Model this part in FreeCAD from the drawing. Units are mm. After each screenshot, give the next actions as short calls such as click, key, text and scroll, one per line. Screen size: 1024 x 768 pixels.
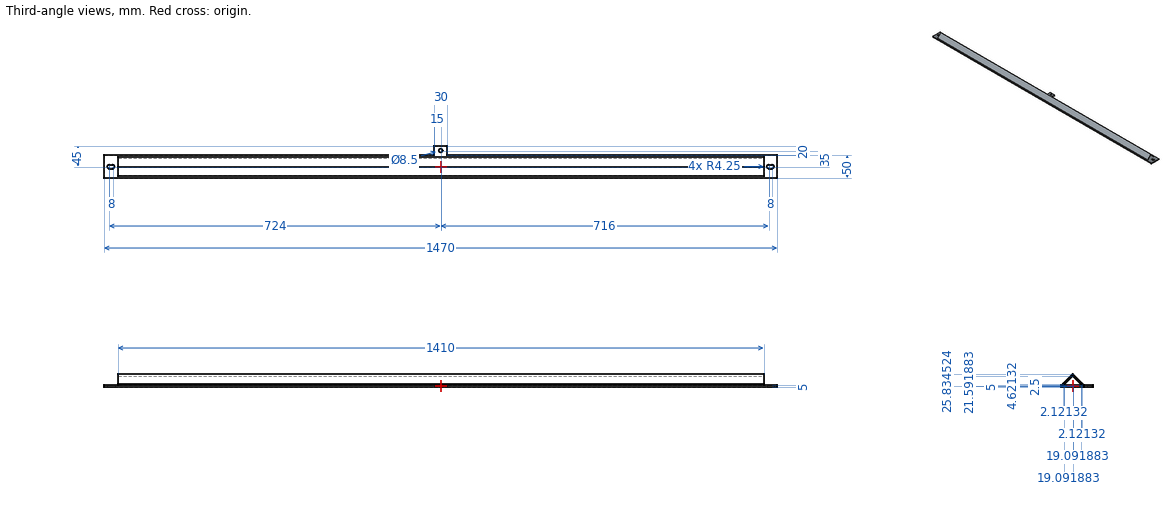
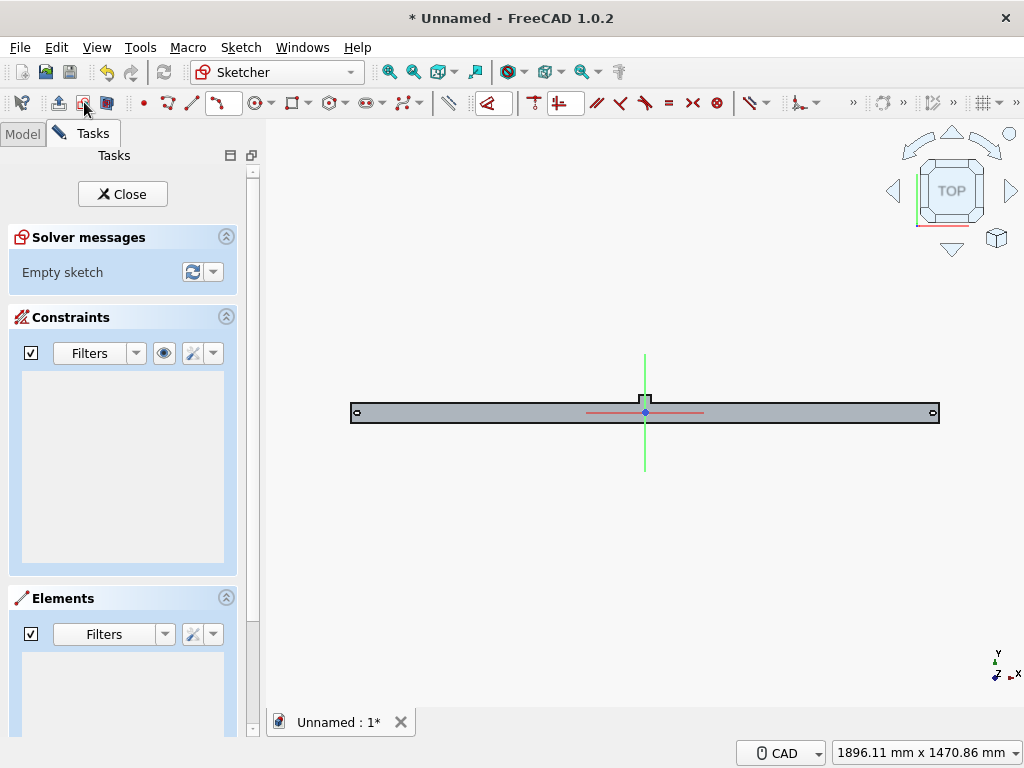
scroll(649, 398, up, 15)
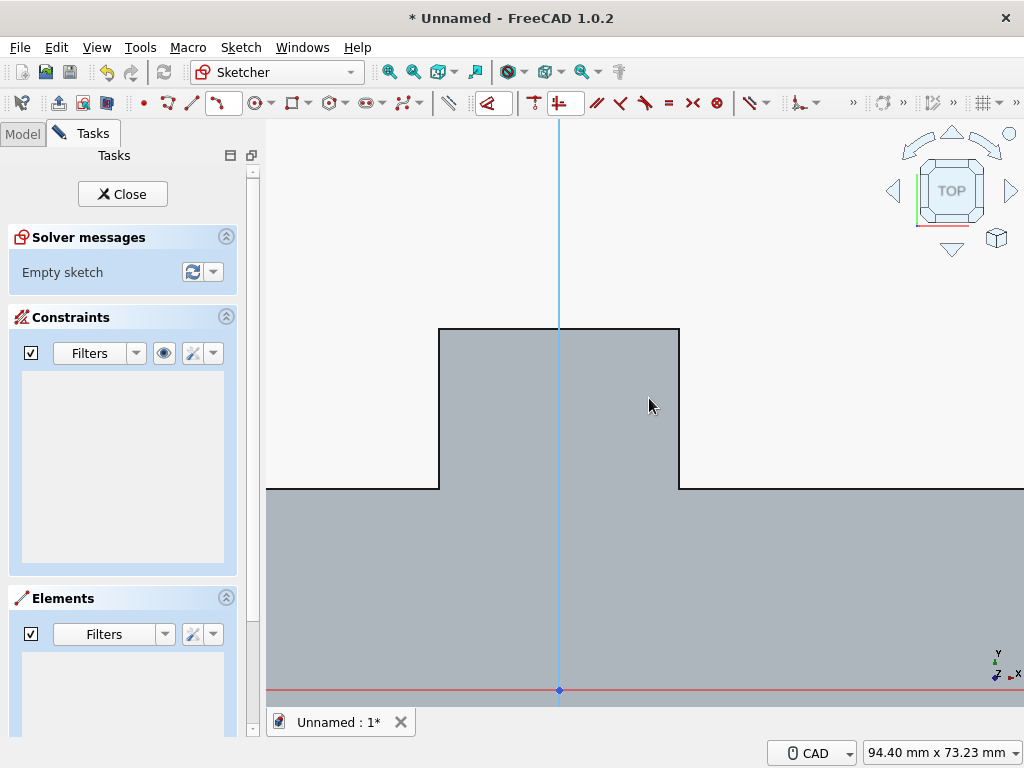
scroll(556, 408, up, 9)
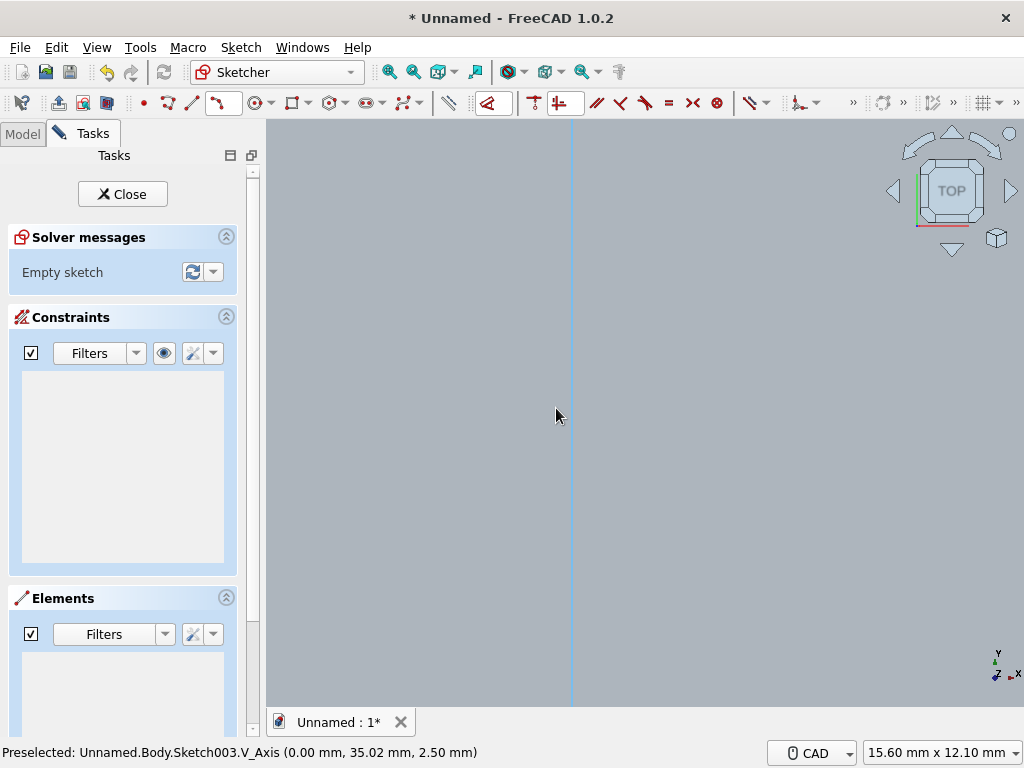
click(256, 104)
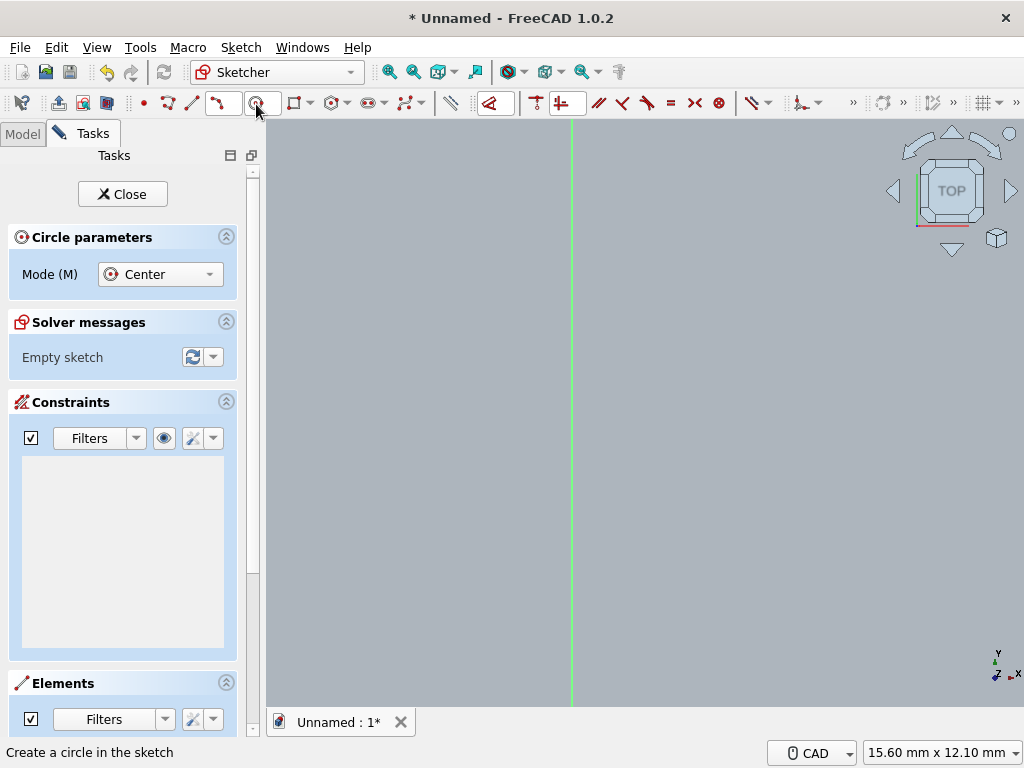
click(572, 413)
move(718, 267)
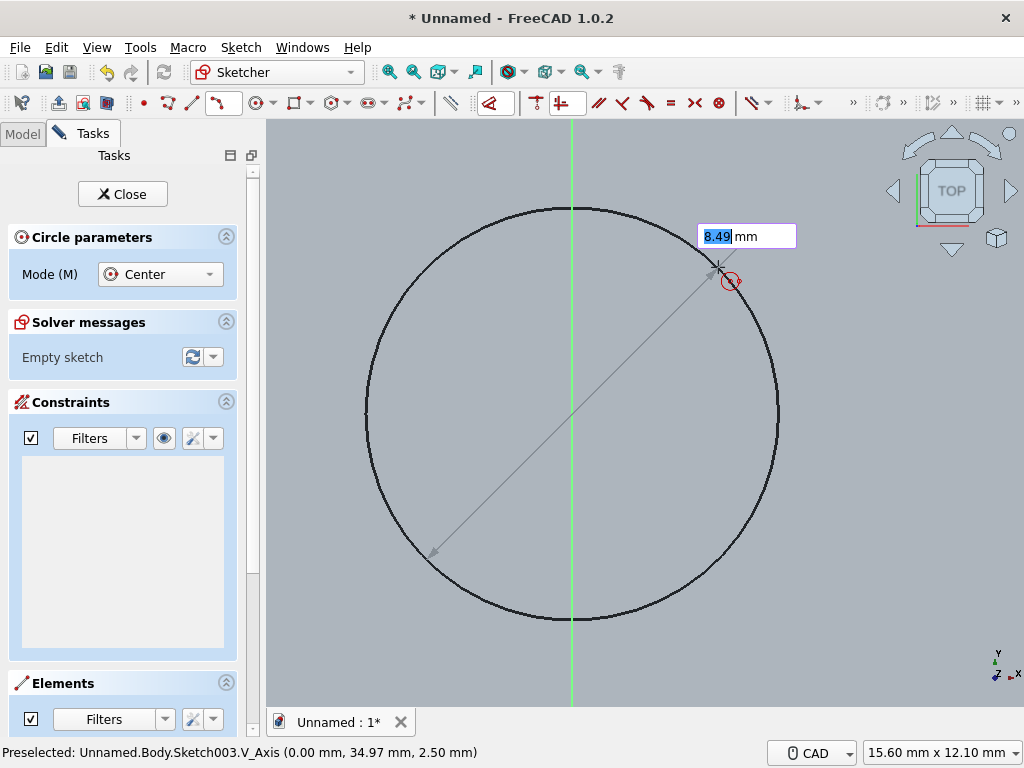
text(8.5)
key(Return)
key(Escape)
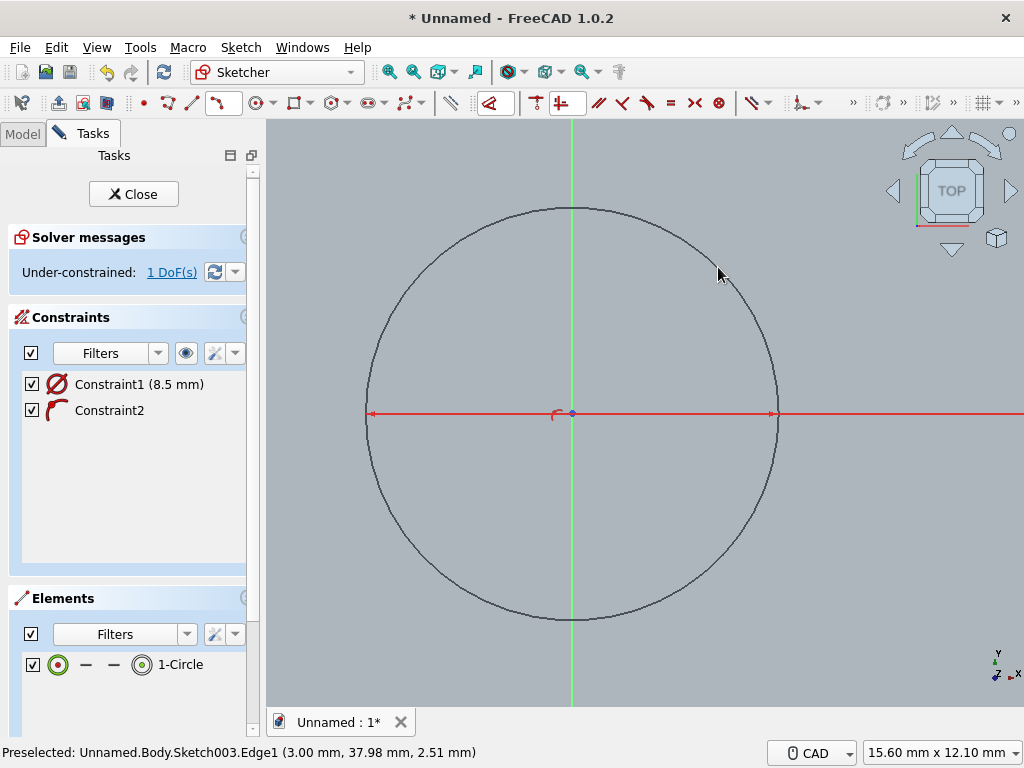
click(572, 414)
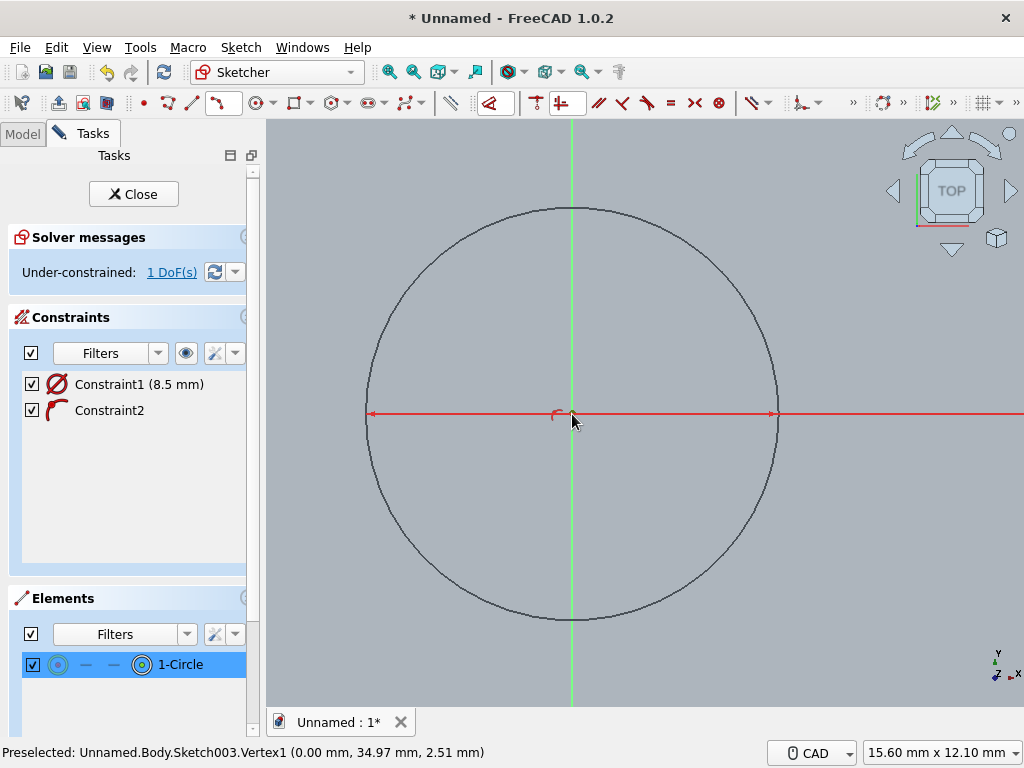
key(i)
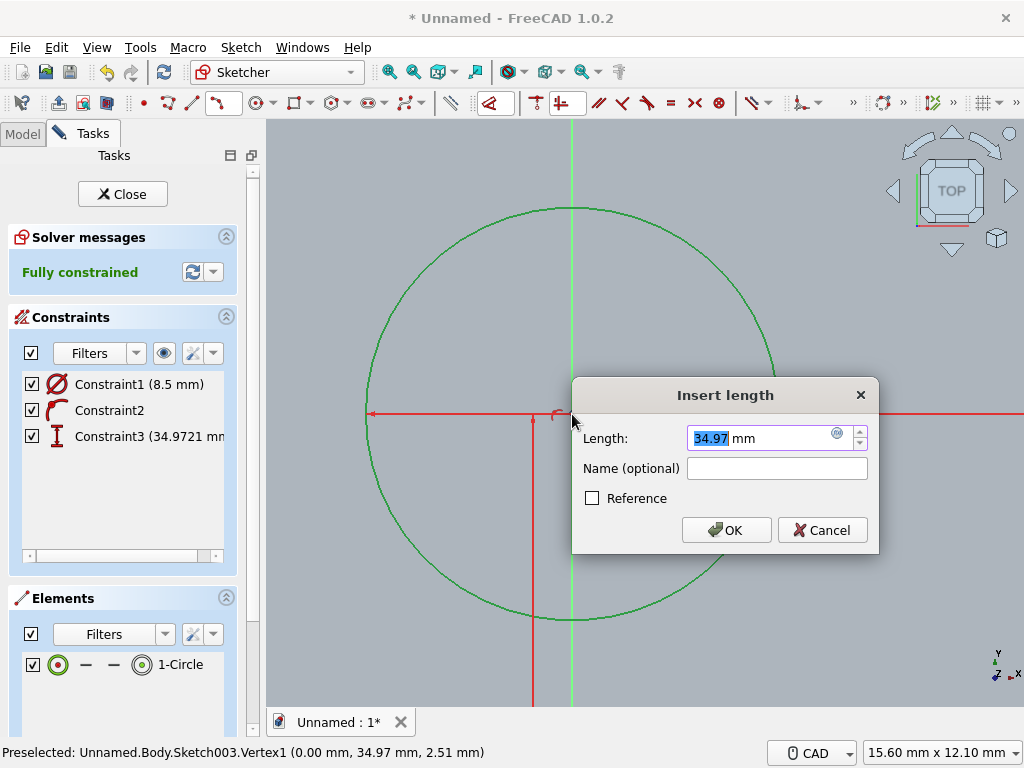
text(35)
key(Return)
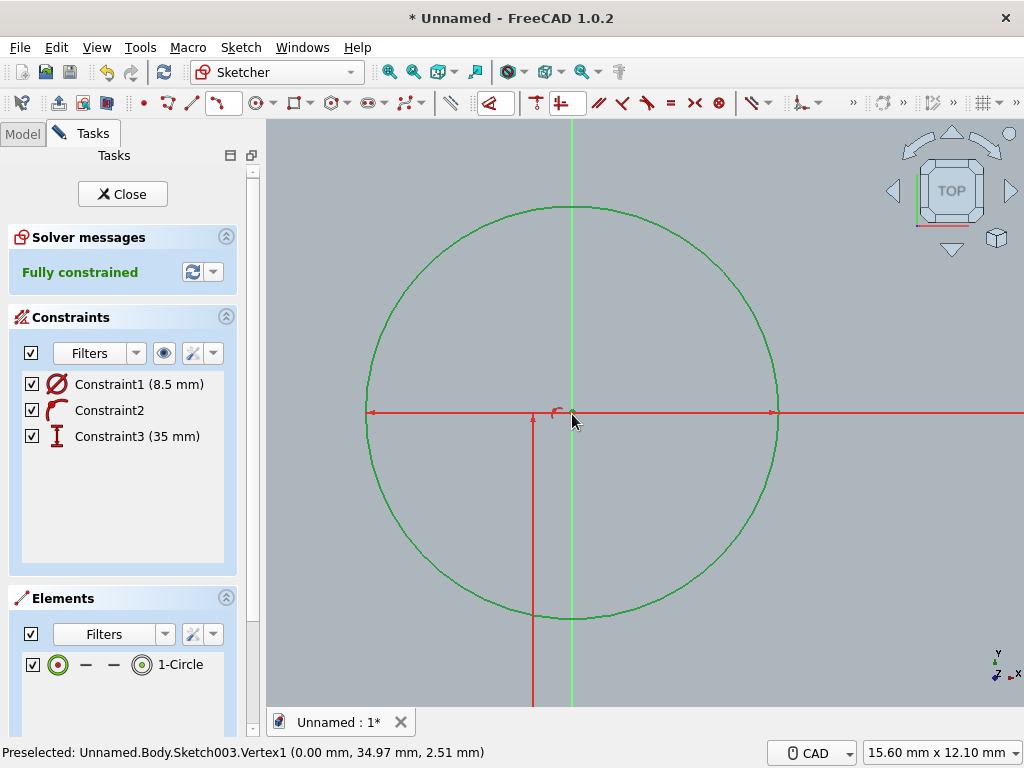
click(123, 194)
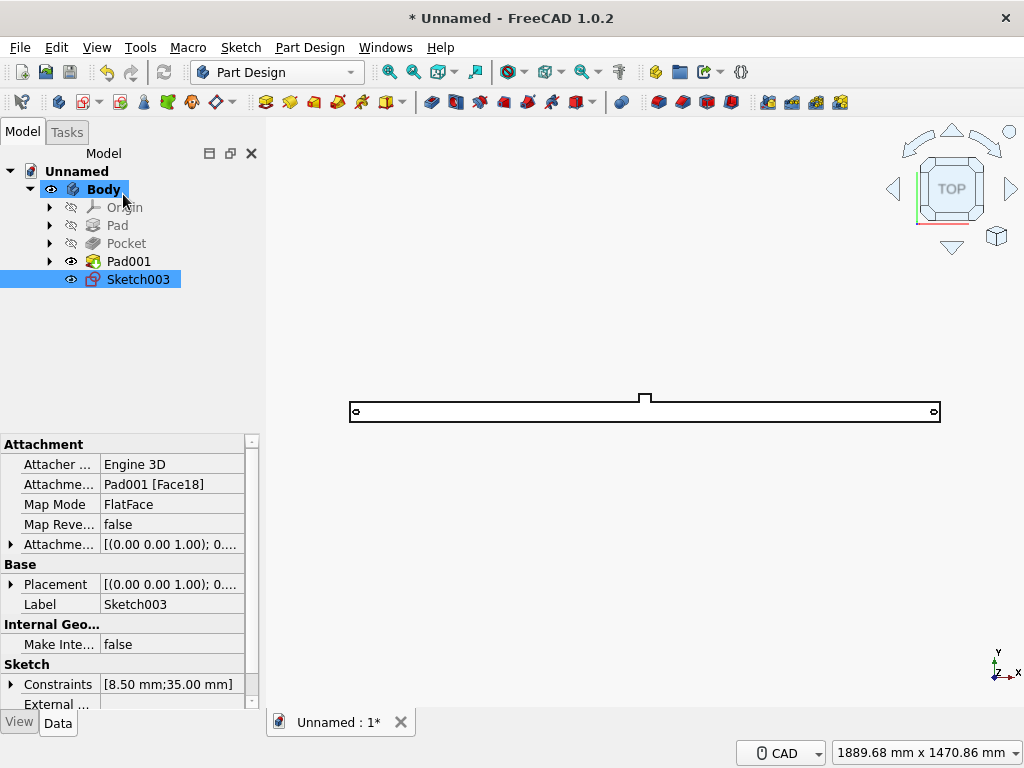
click(432, 102)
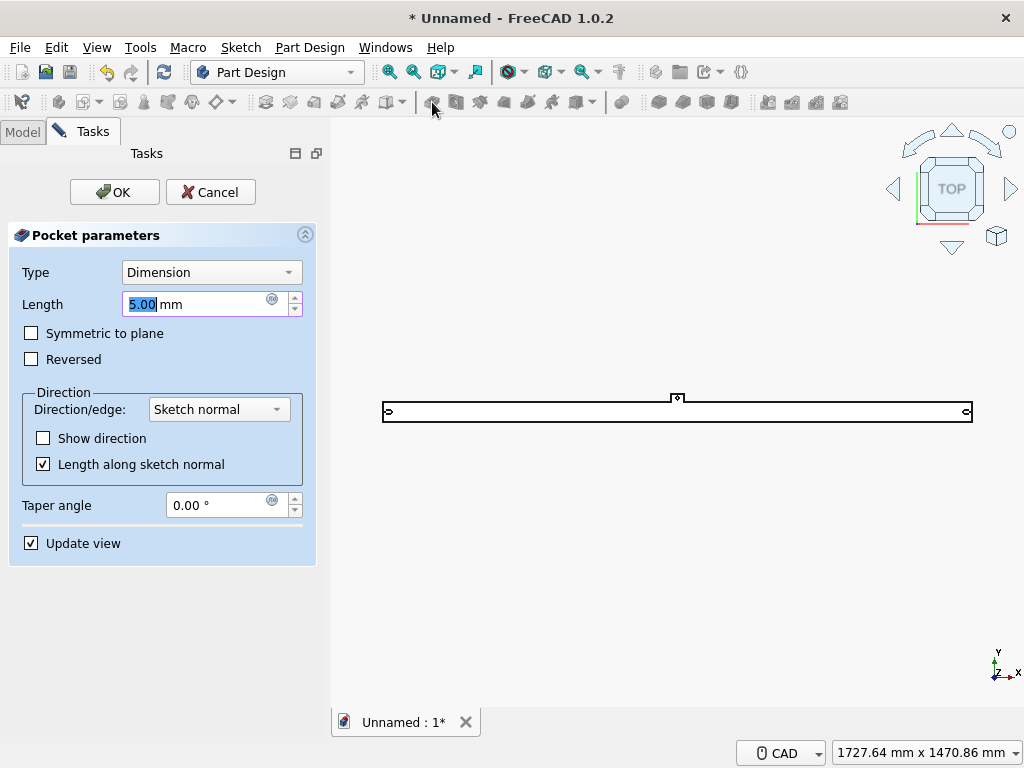
text(5)
key(Tab)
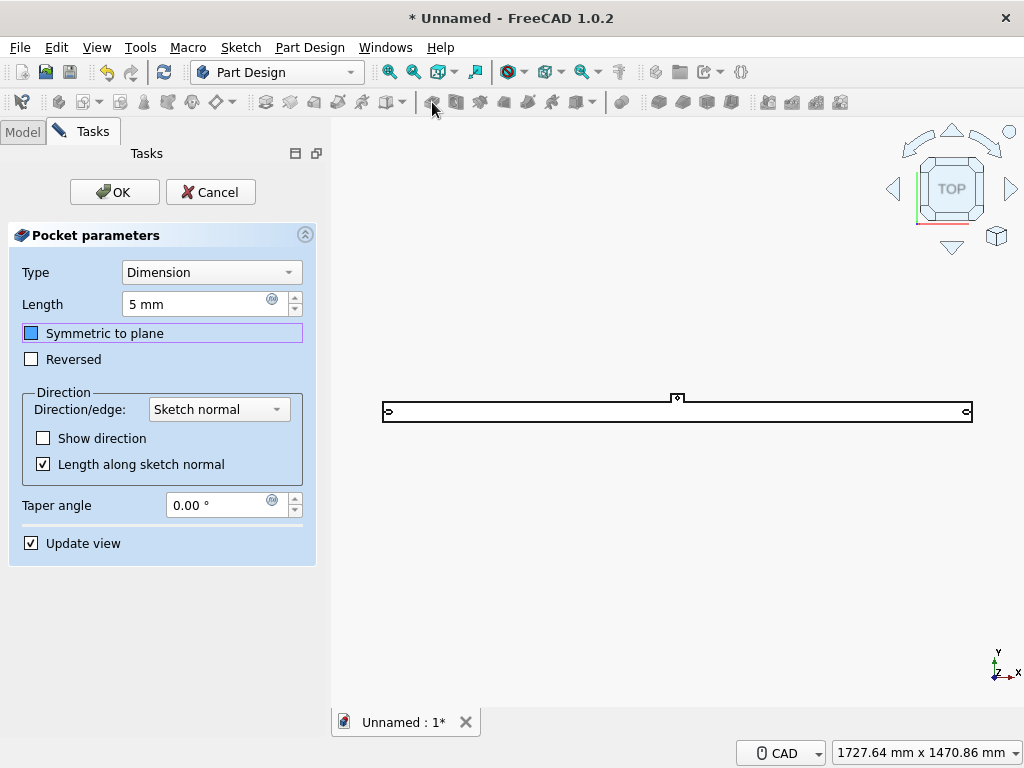
click(115, 192)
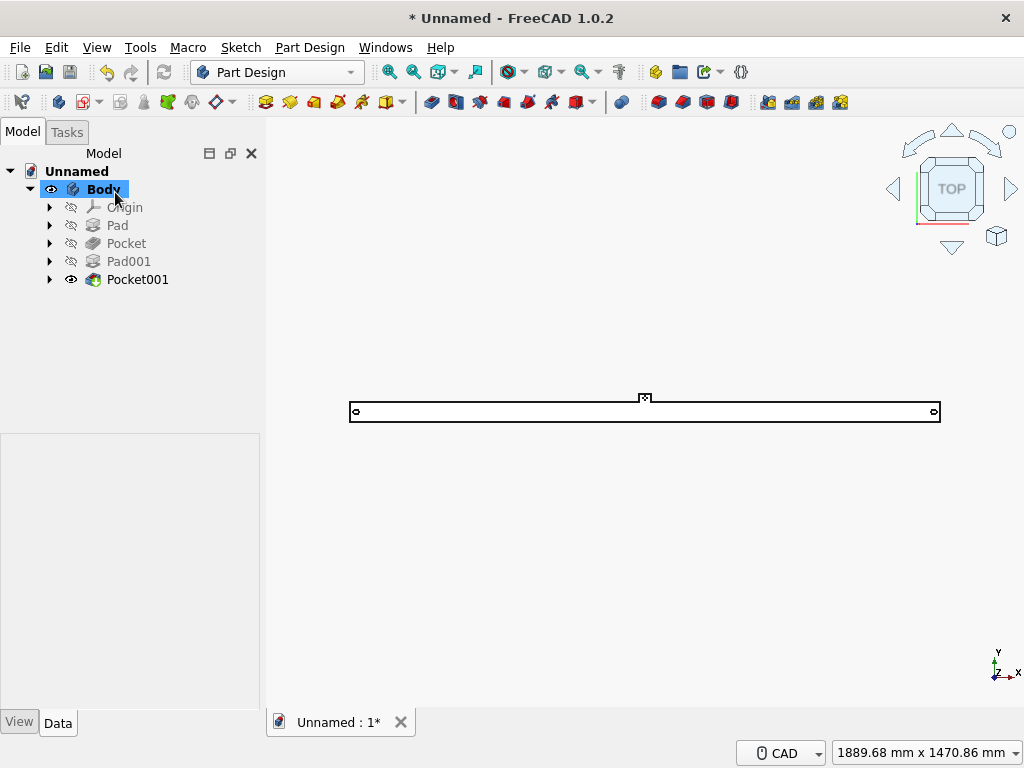
click(60, 102)